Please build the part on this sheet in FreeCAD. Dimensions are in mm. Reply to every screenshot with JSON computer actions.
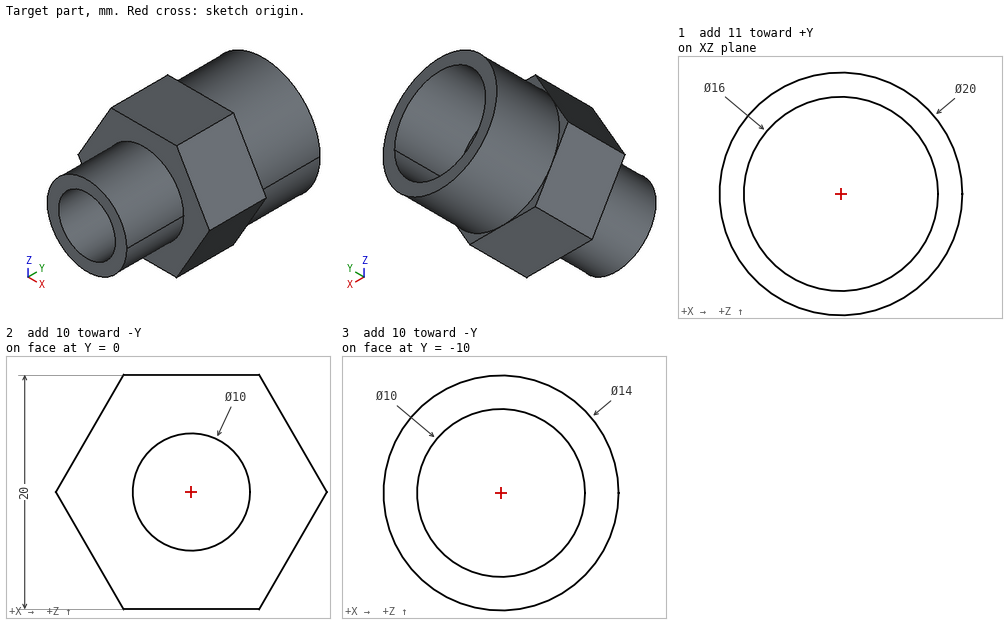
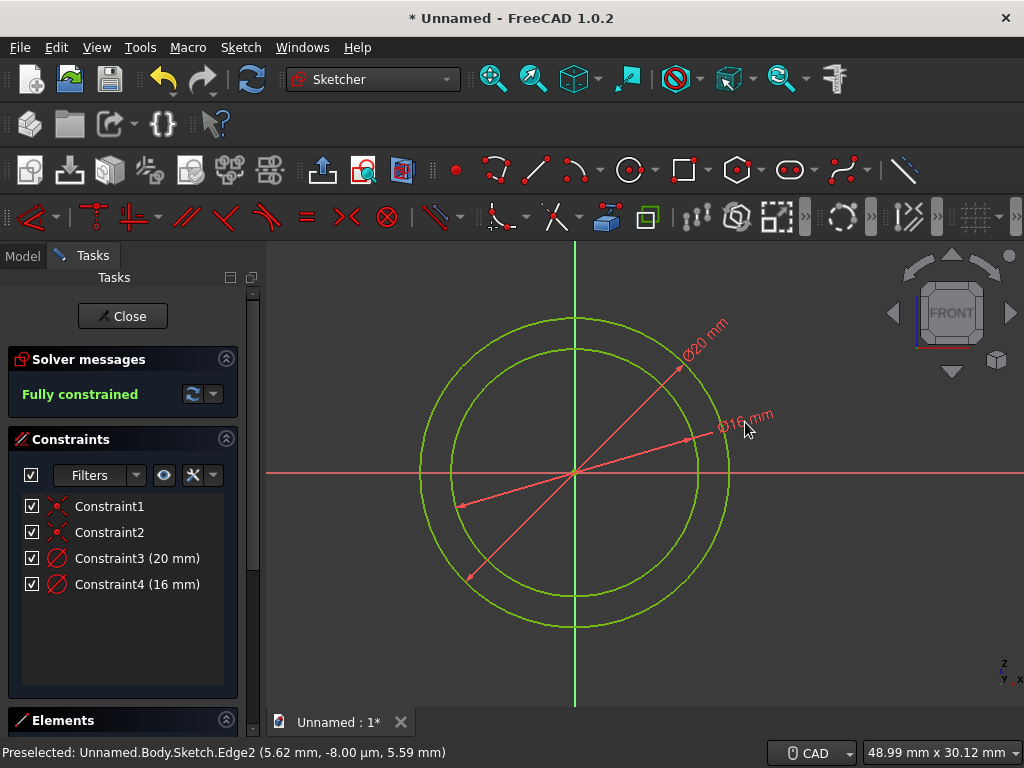
{"action": "left_click", "coordinate": [123, 316]}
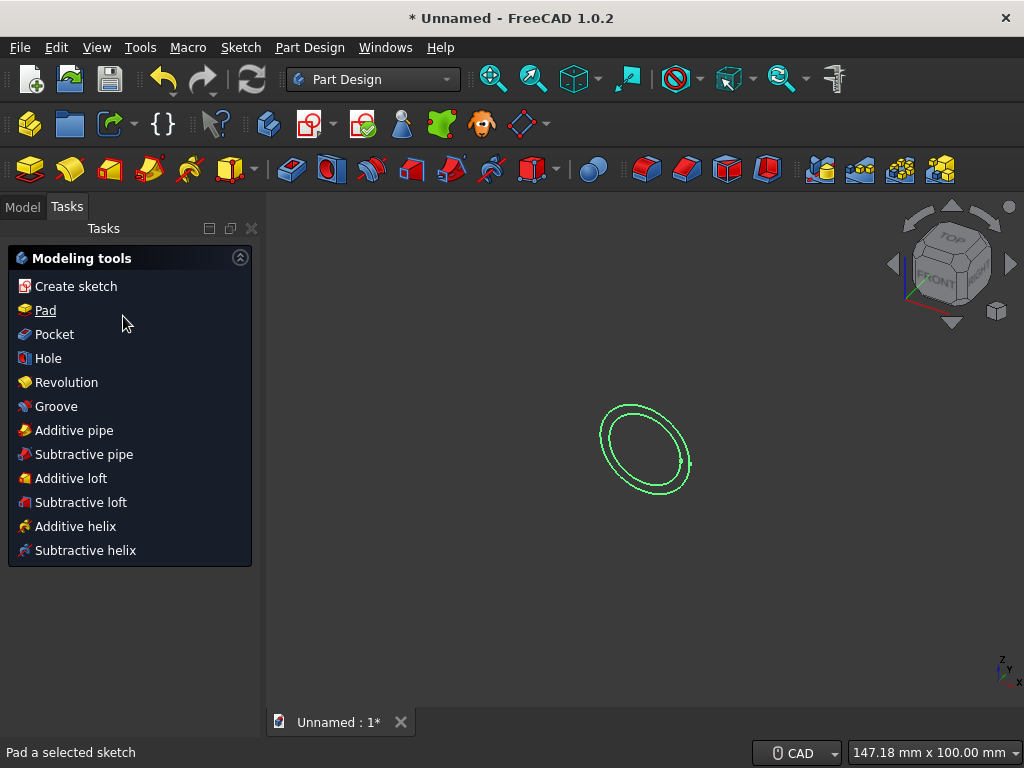
{"action": "left_click", "coordinate": [30, 170]}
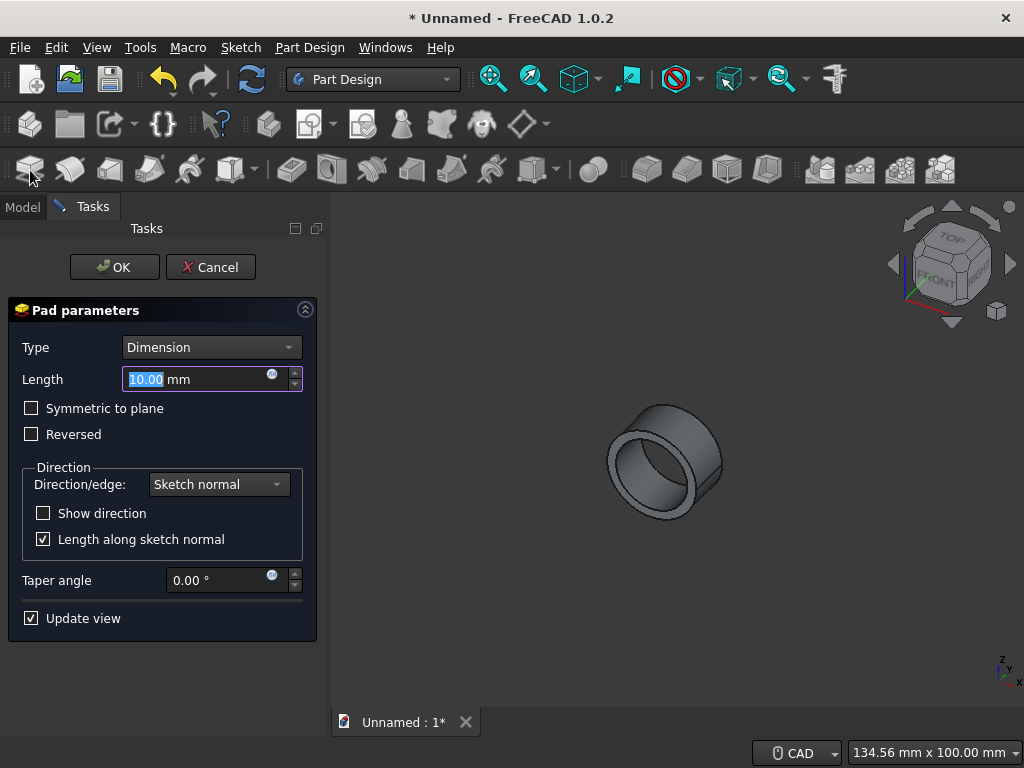
{"action": "type", "text": "11"}
{"action": "key", "text": "Tab"}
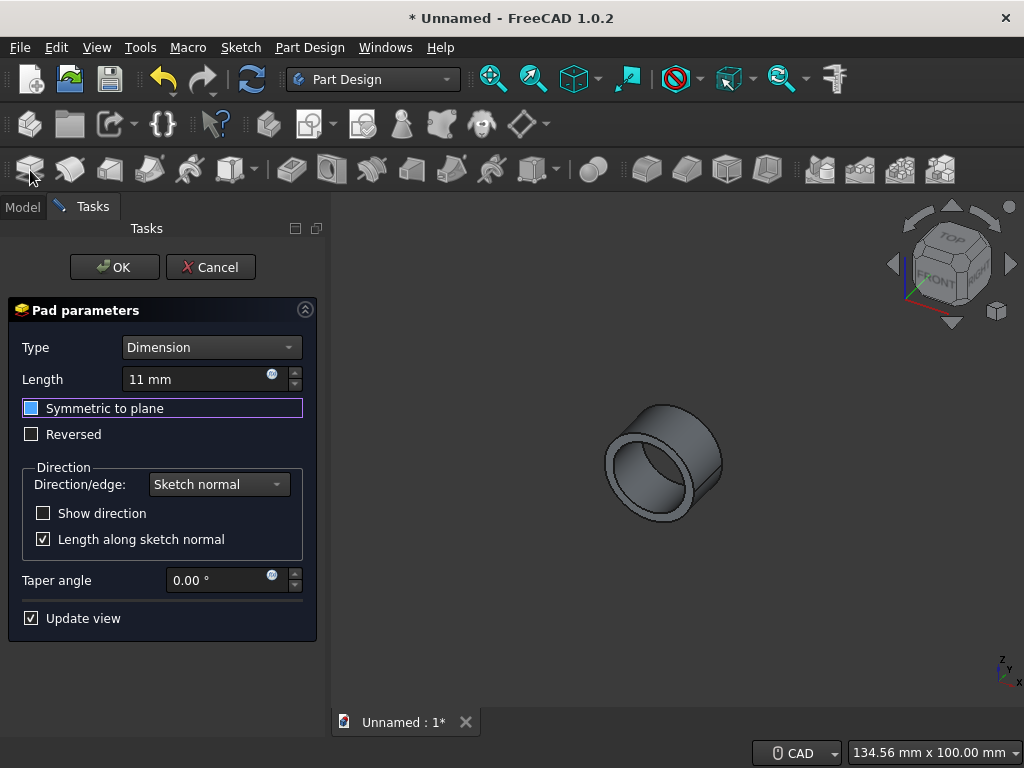
{"action": "left_click", "coordinate": [30, 434]}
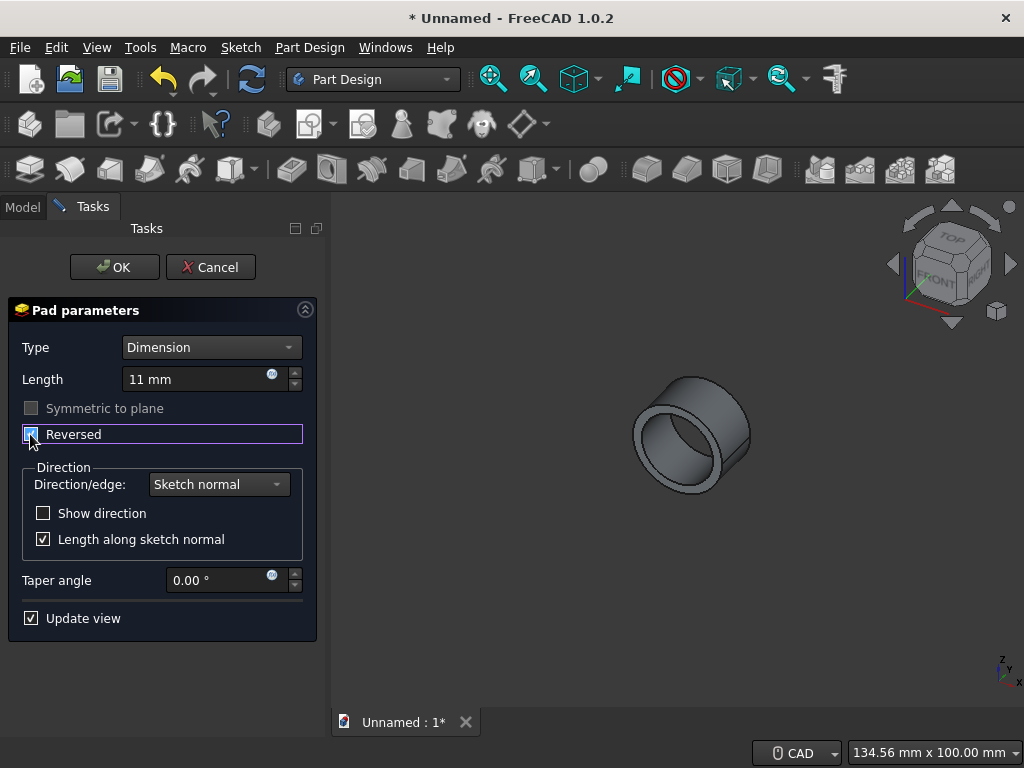
{"action": "left_click", "coordinate": [115, 267]}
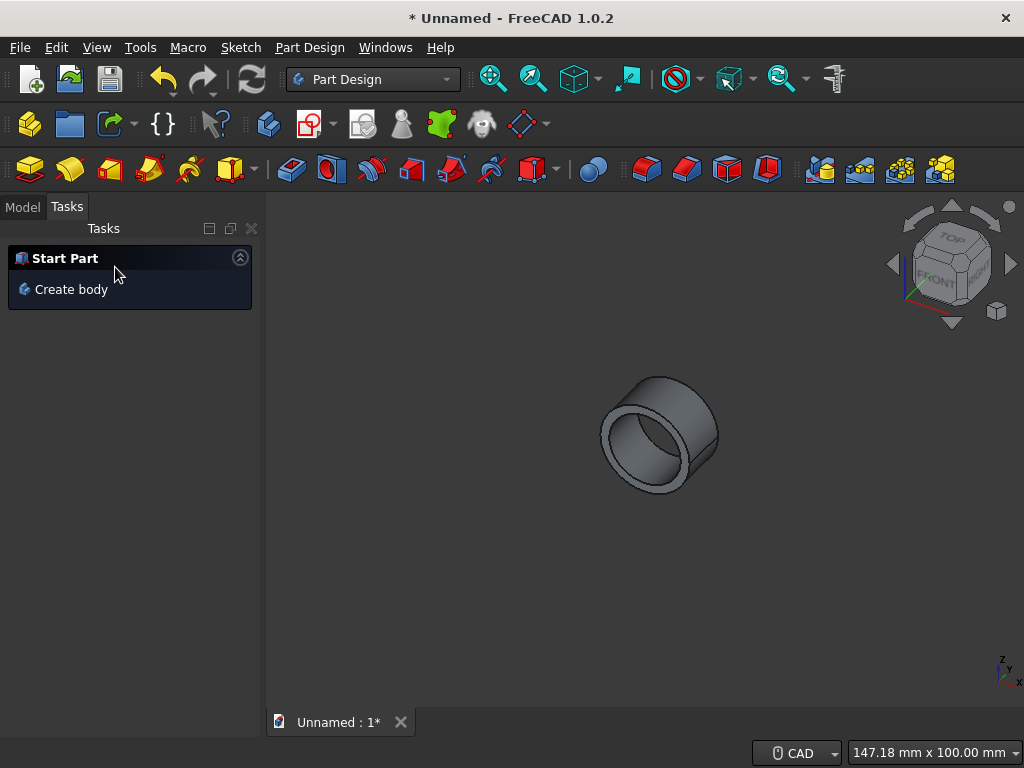
{"action": "left_click", "coordinate": [494, 80]}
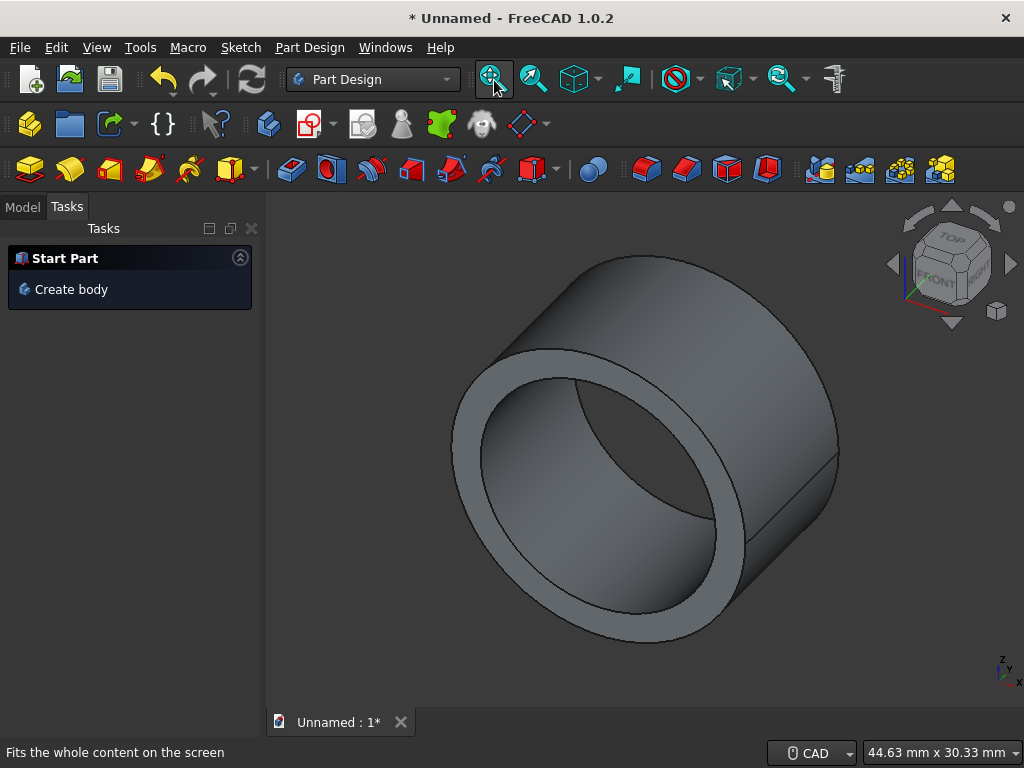
{"action": "left_click", "coordinate": [556, 600]}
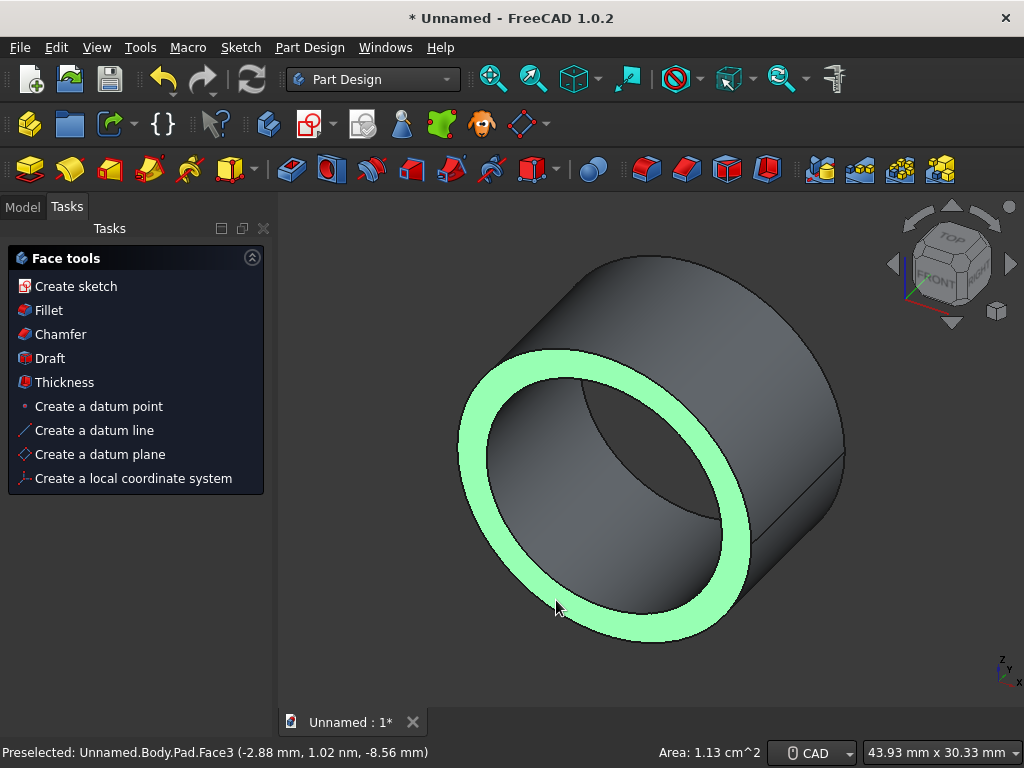
{"action": "left_click", "coordinate": [310, 124]}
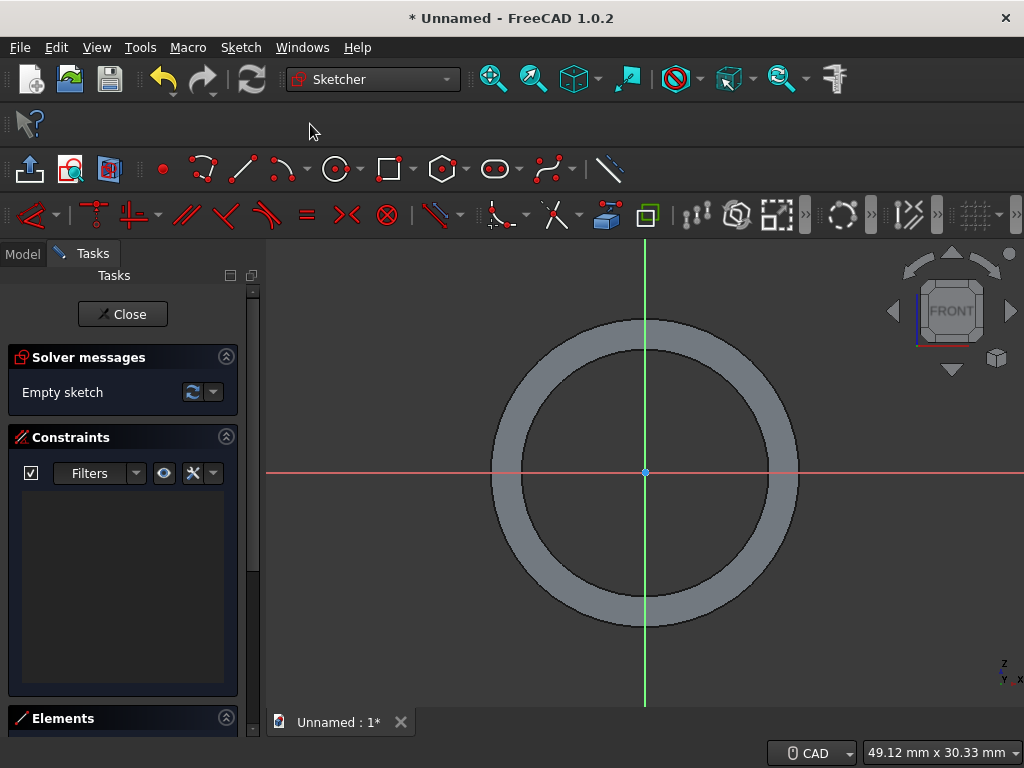
{"action": "left_click", "coordinate": [442, 170]}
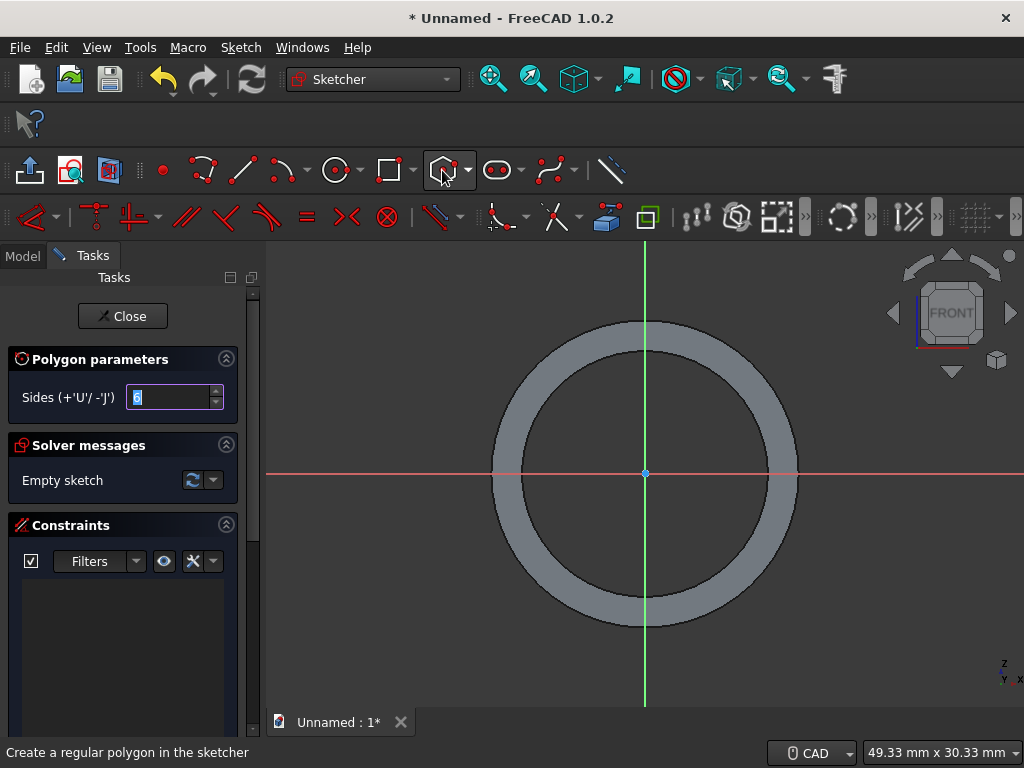
{"action": "left_click", "coordinate": [645, 474]}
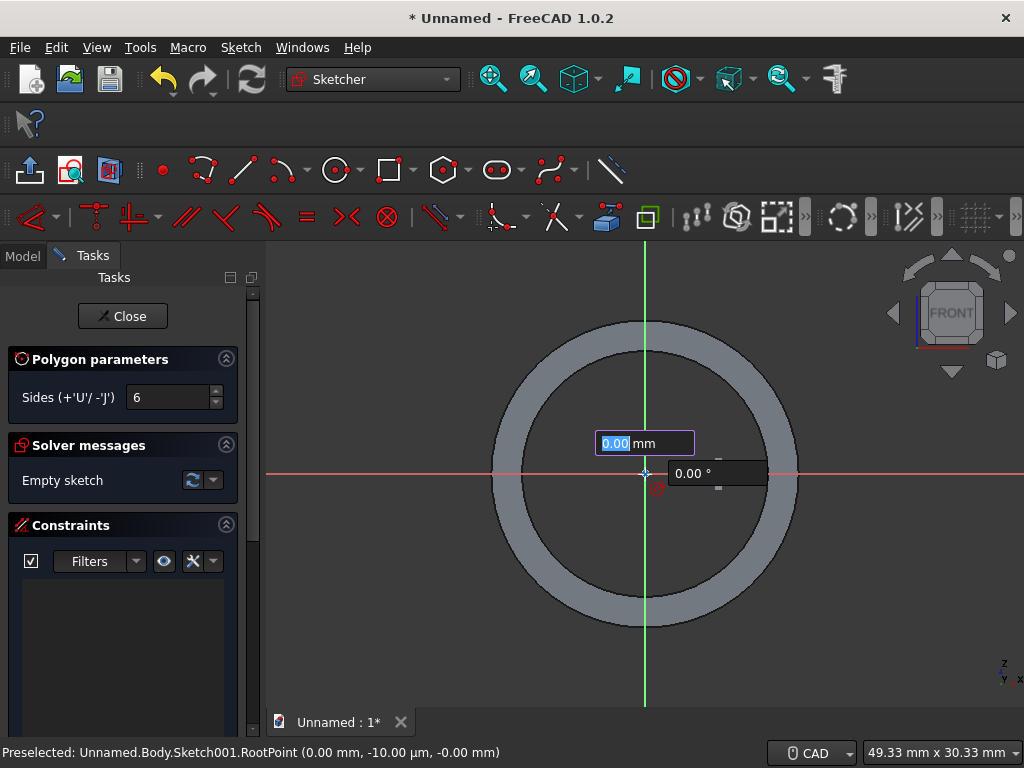
{"action": "left_click", "coordinate": [822, 474]}
{"action": "right_click", "coordinate": [822, 474]}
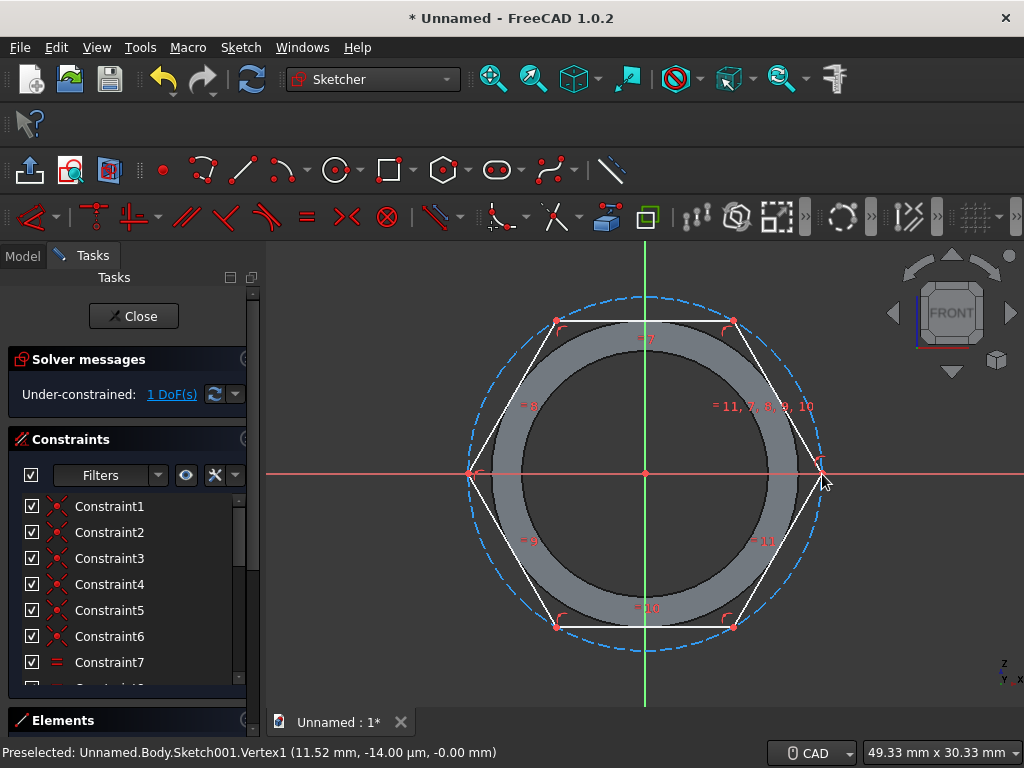
{"action": "left_click", "coordinate": [336, 170]}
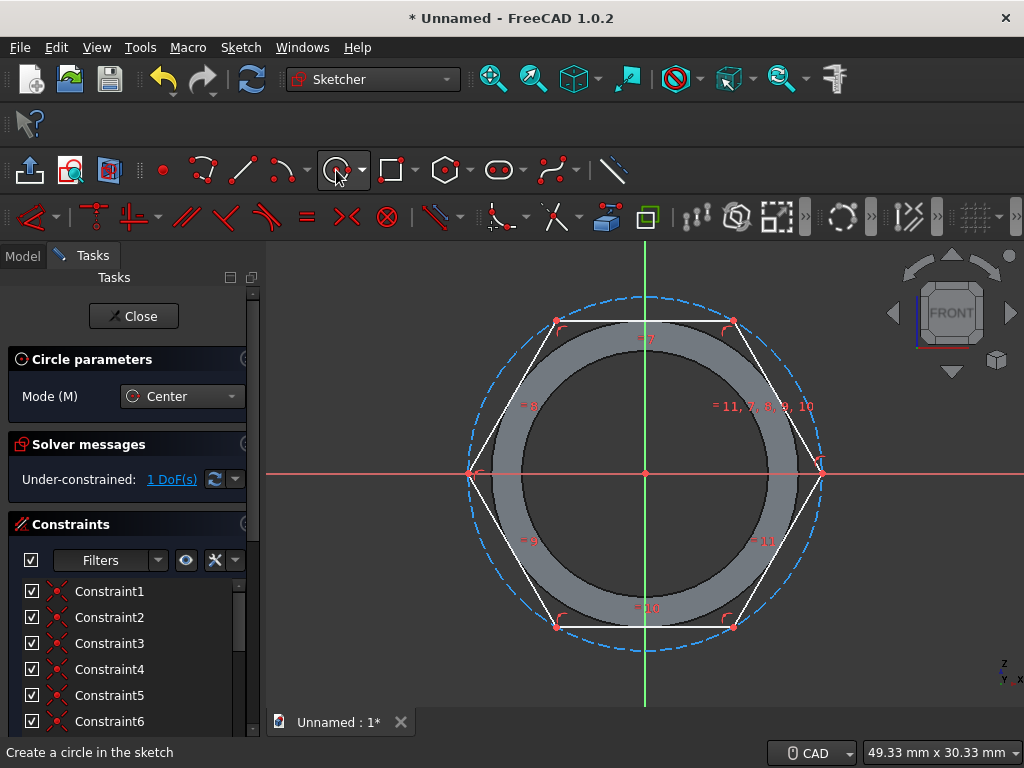
{"action": "left_click", "coordinate": [645, 474]}
{"action": "left_click", "coordinate": [699, 420]}
{"action": "key", "text": "Escape"}